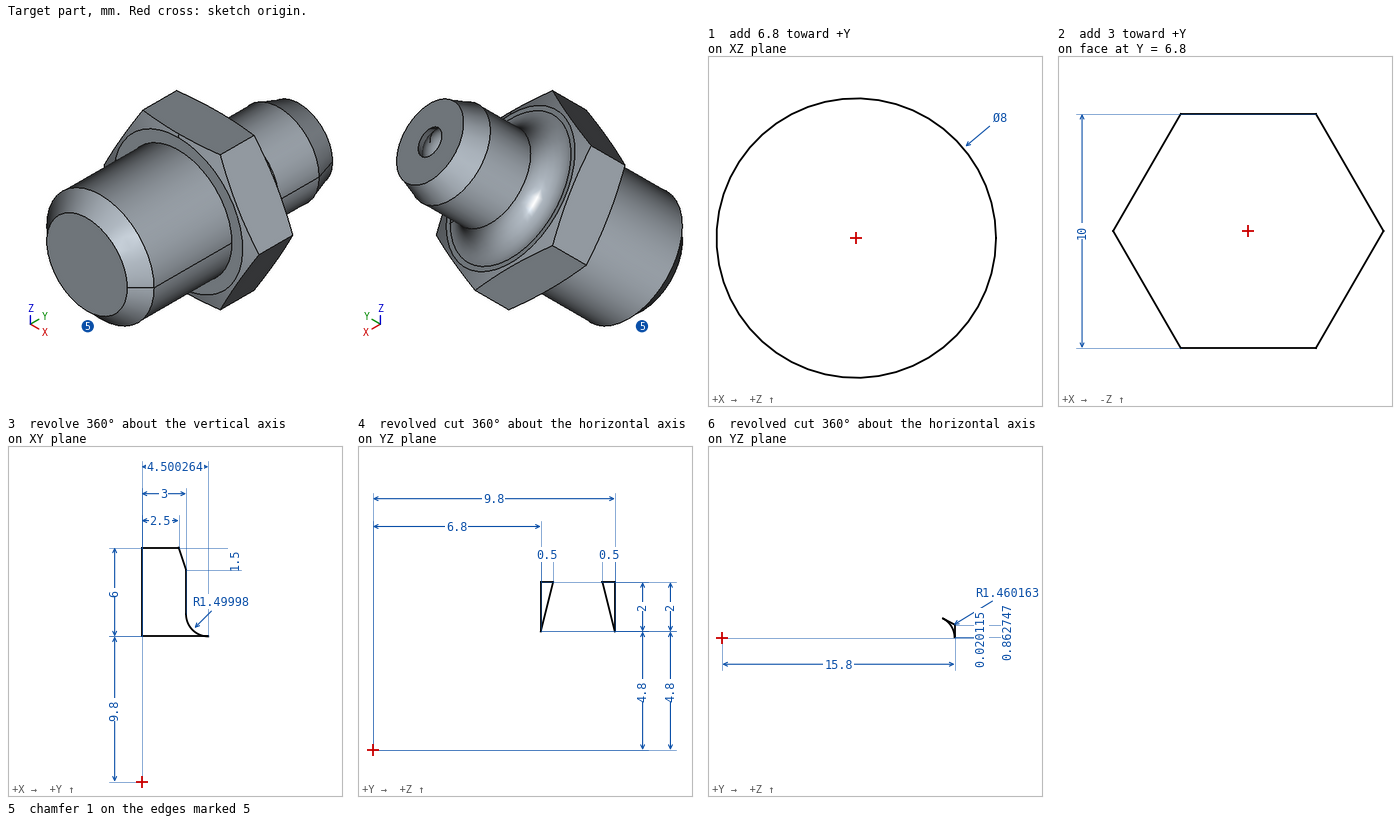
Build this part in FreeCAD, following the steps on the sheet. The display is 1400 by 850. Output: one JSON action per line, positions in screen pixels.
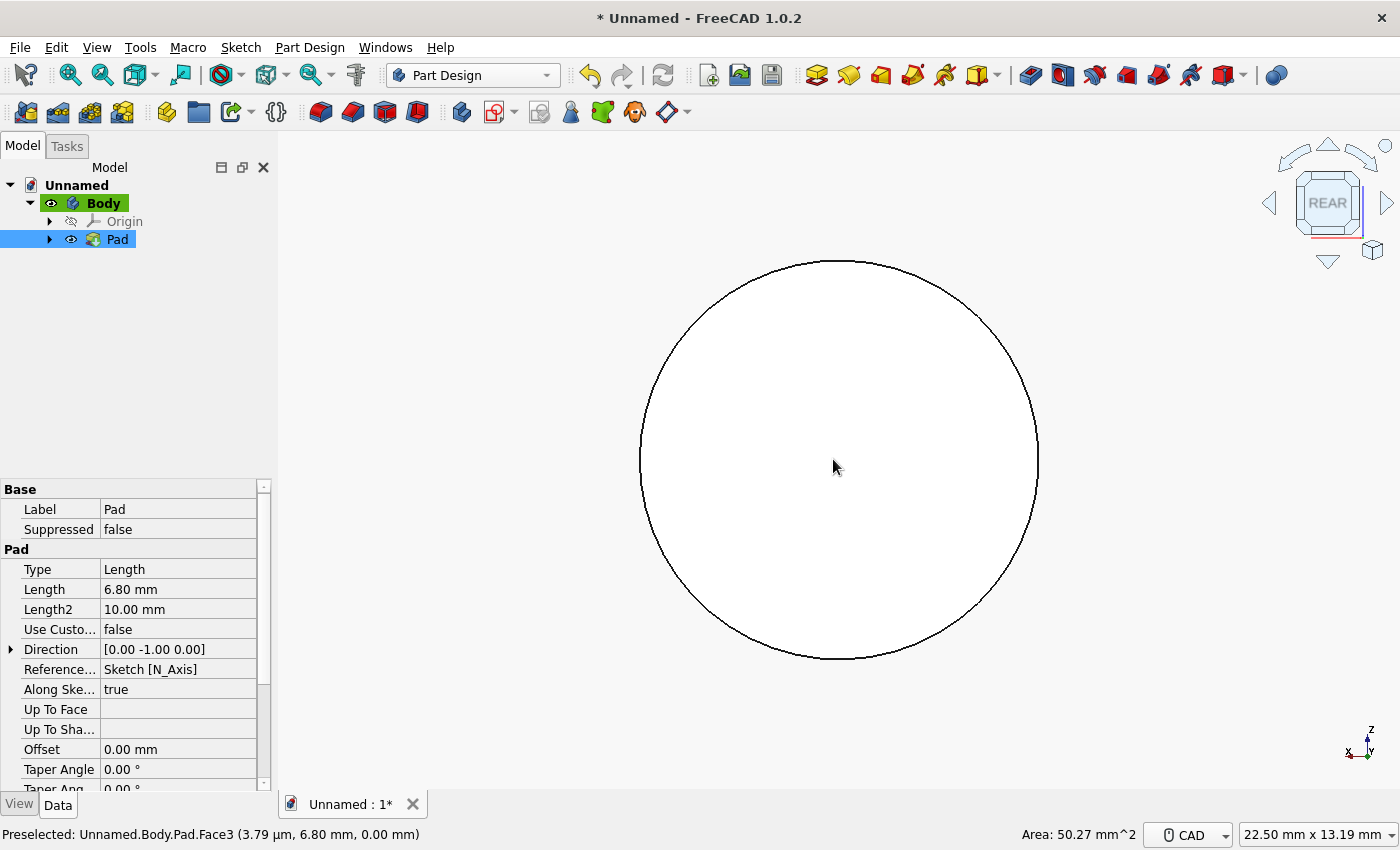
{"action": "left_click", "coordinate": [494, 112]}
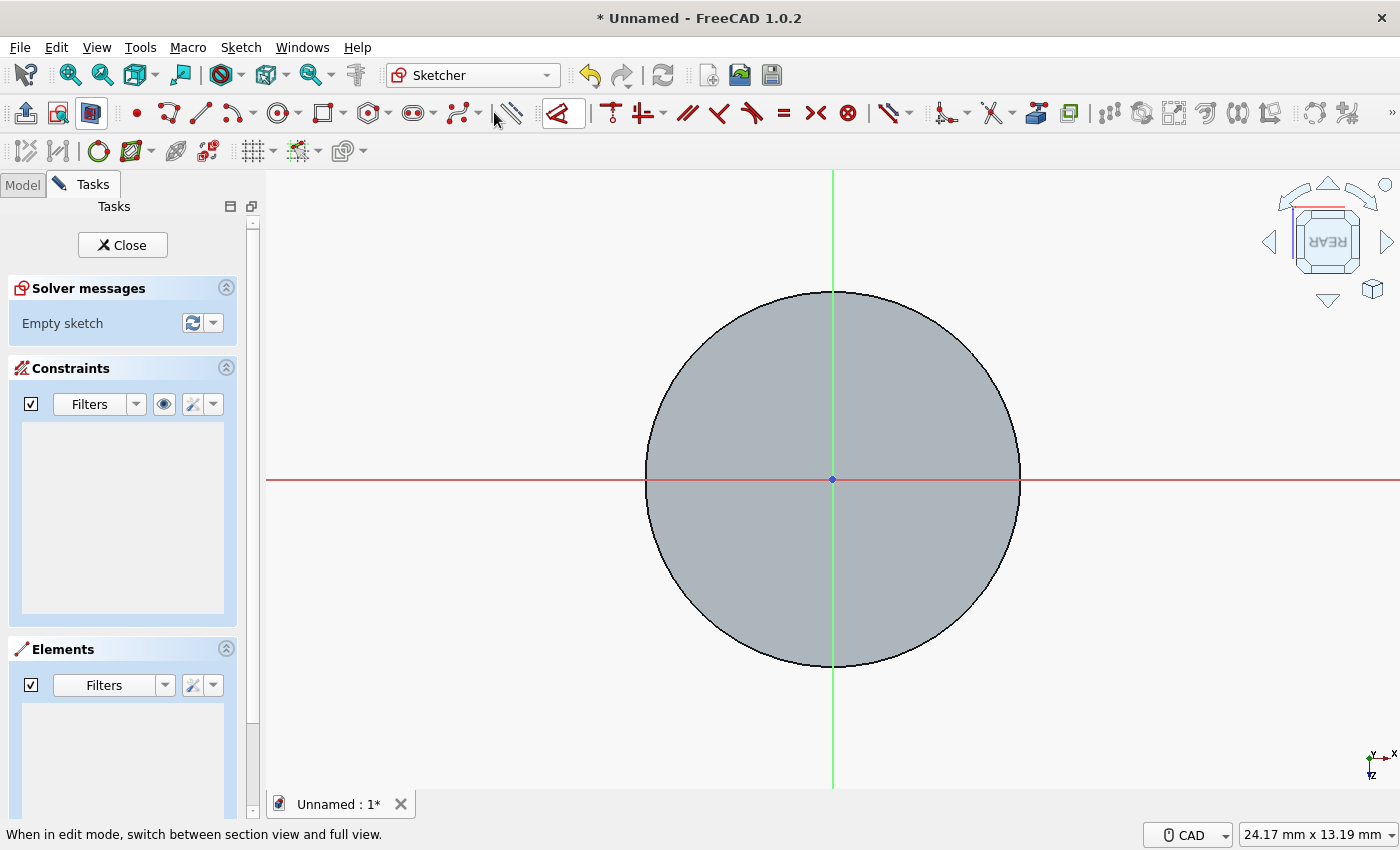
{"action": "left_click", "coordinate": [368, 114]}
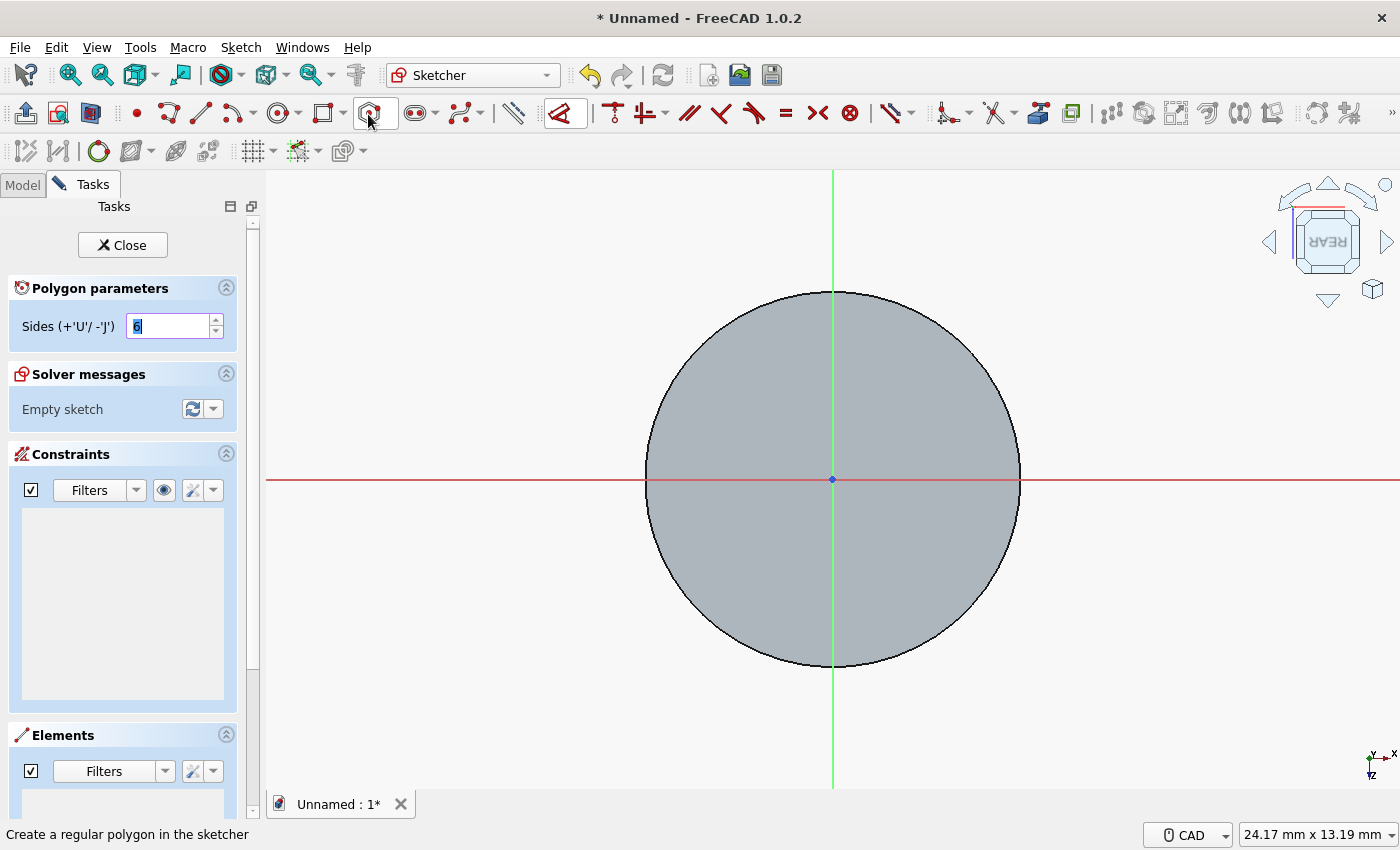
{"action": "left_click", "coordinate": [833, 479]}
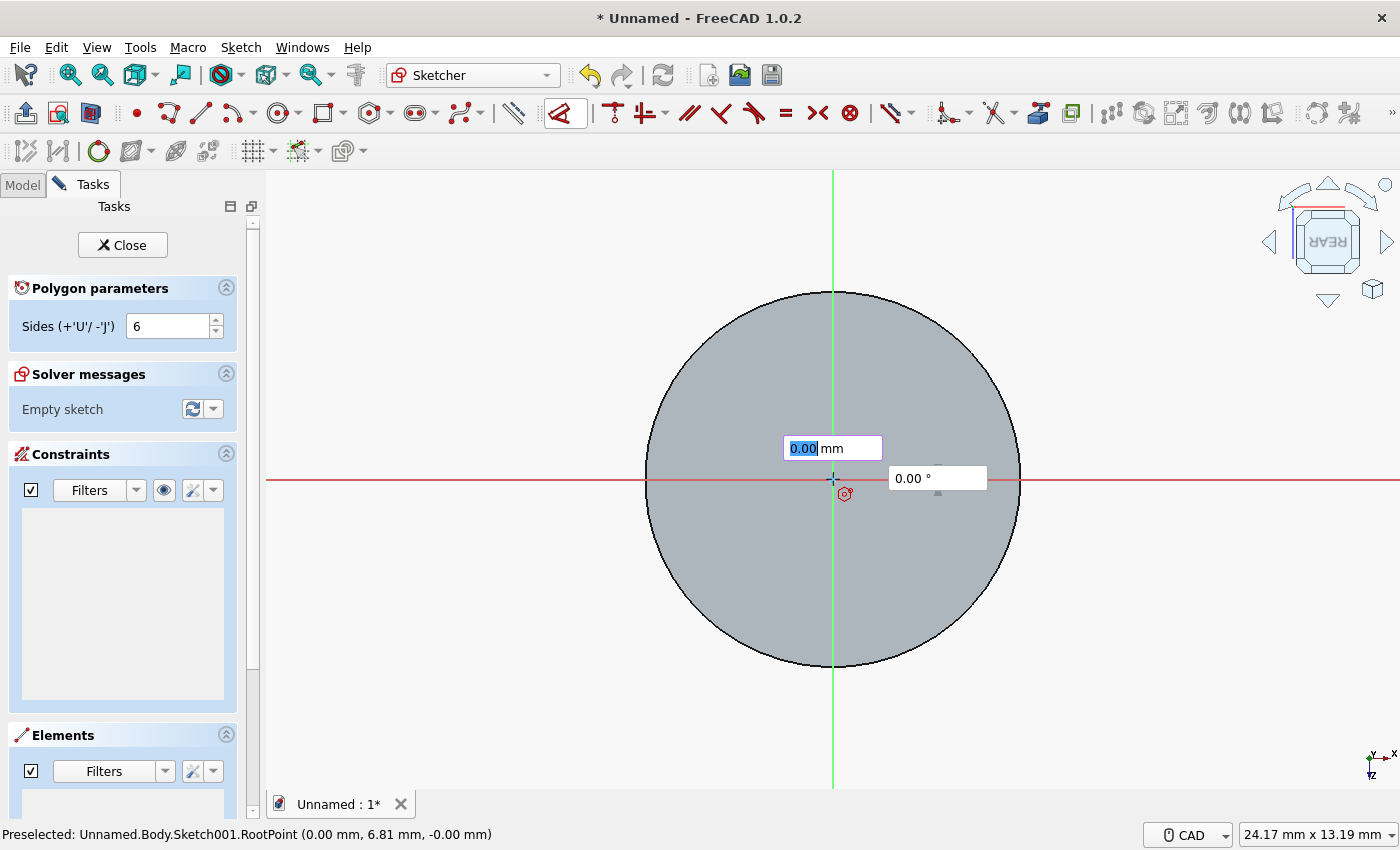
{"action": "left_click", "coordinate": [1104, 479]}
{"action": "right_click", "coordinate": [1104, 479]}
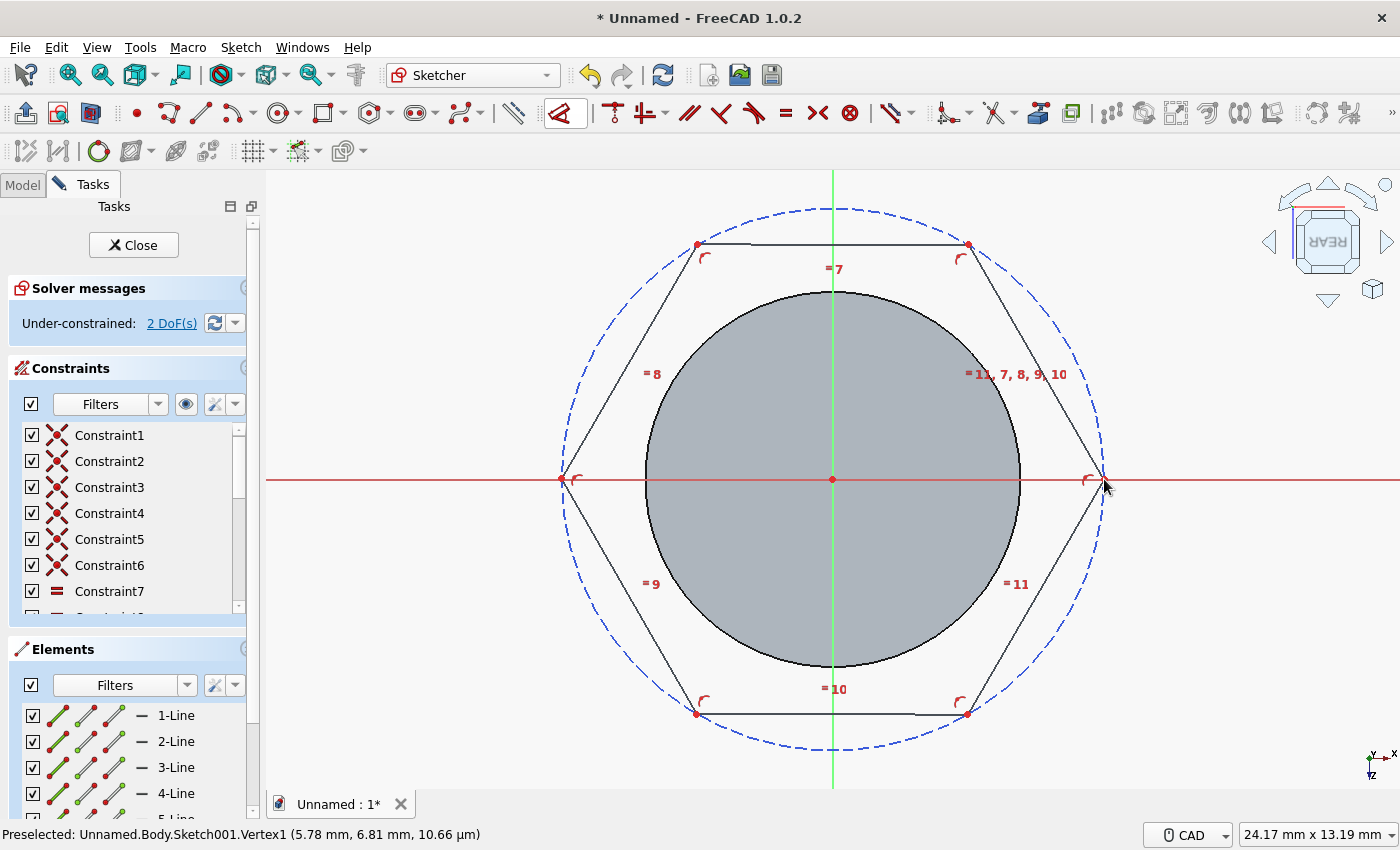
{"action": "left_click", "coordinate": [887, 245]}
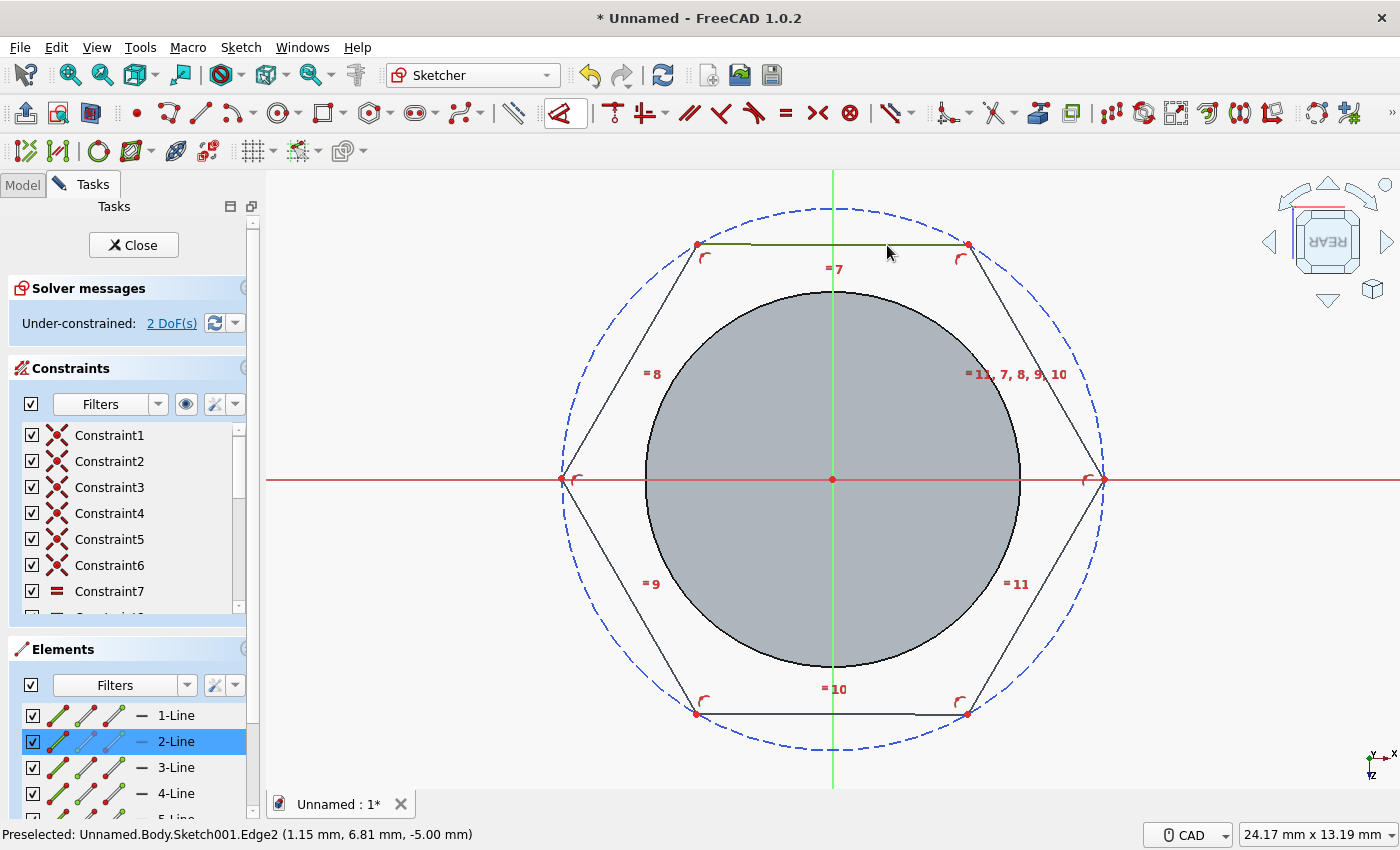
{"action": "key", "text": "h"}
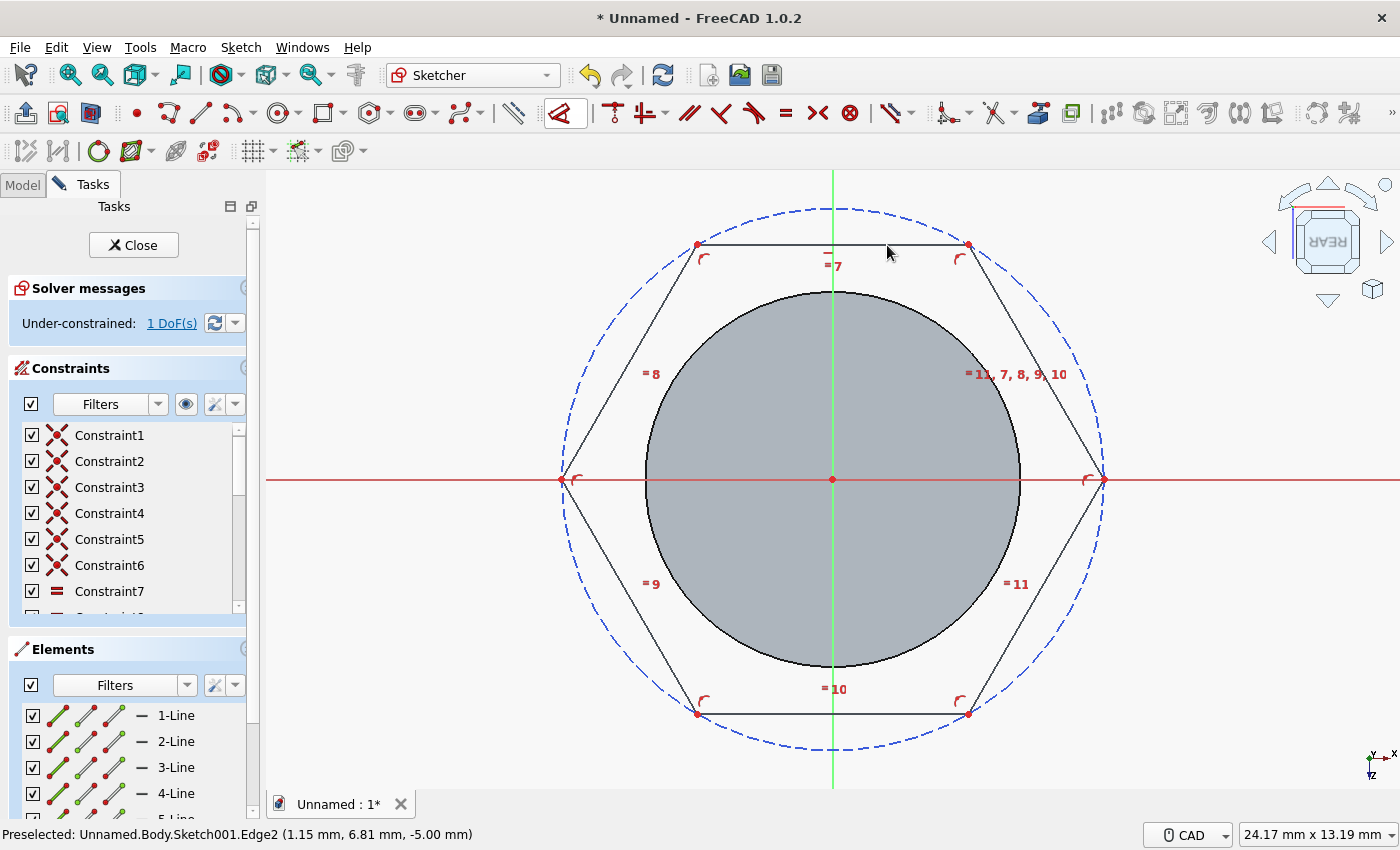
{"action": "left_click", "coordinate": [697, 714]}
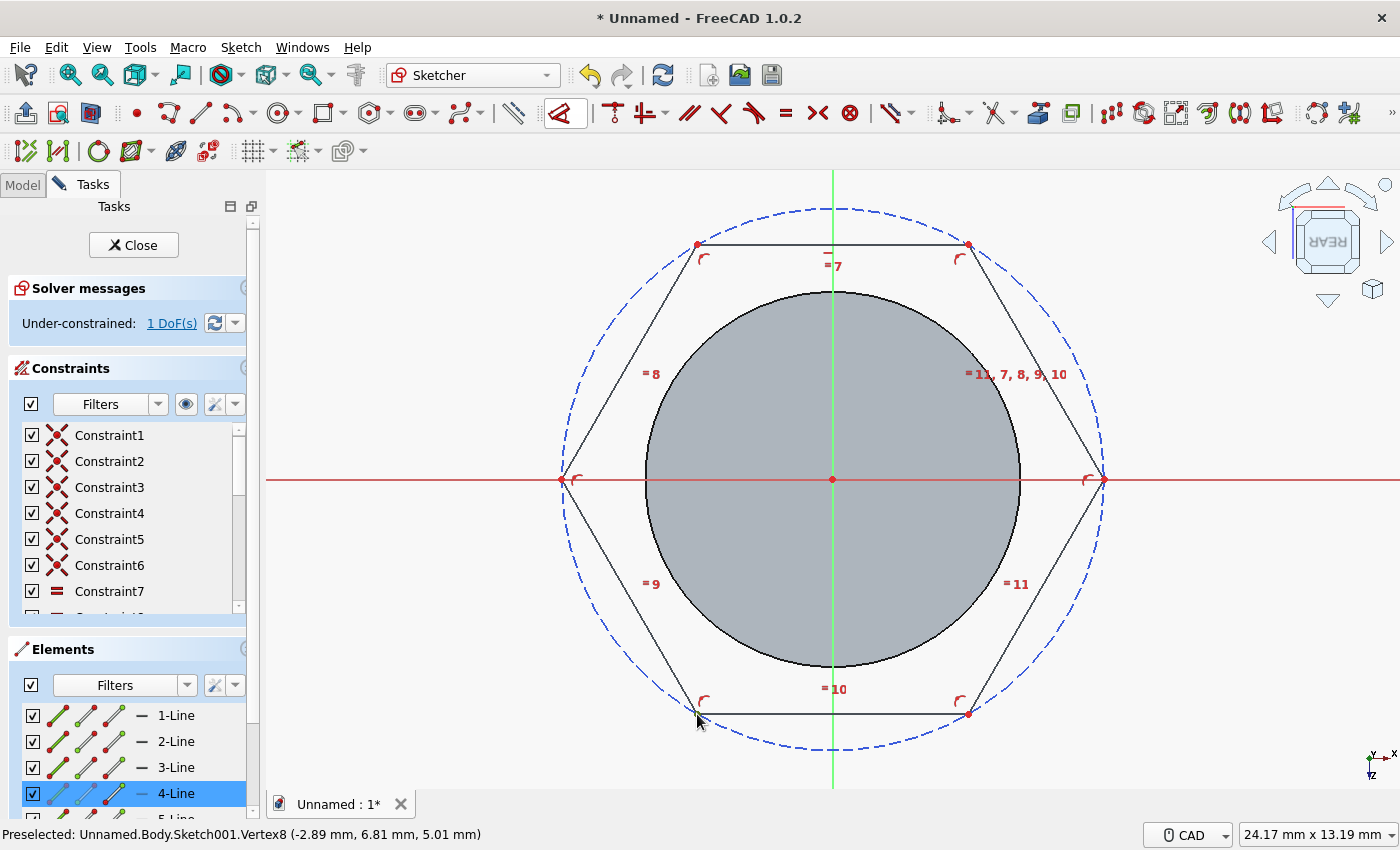
{"action": "left_click", "coordinate": [968, 245]}